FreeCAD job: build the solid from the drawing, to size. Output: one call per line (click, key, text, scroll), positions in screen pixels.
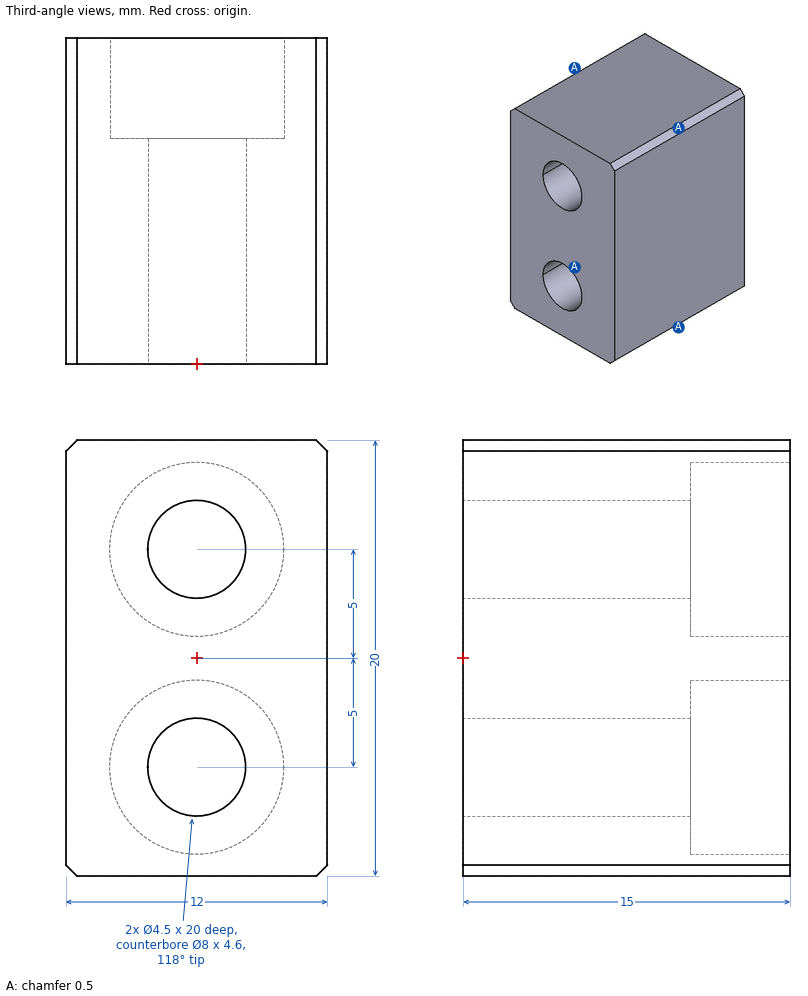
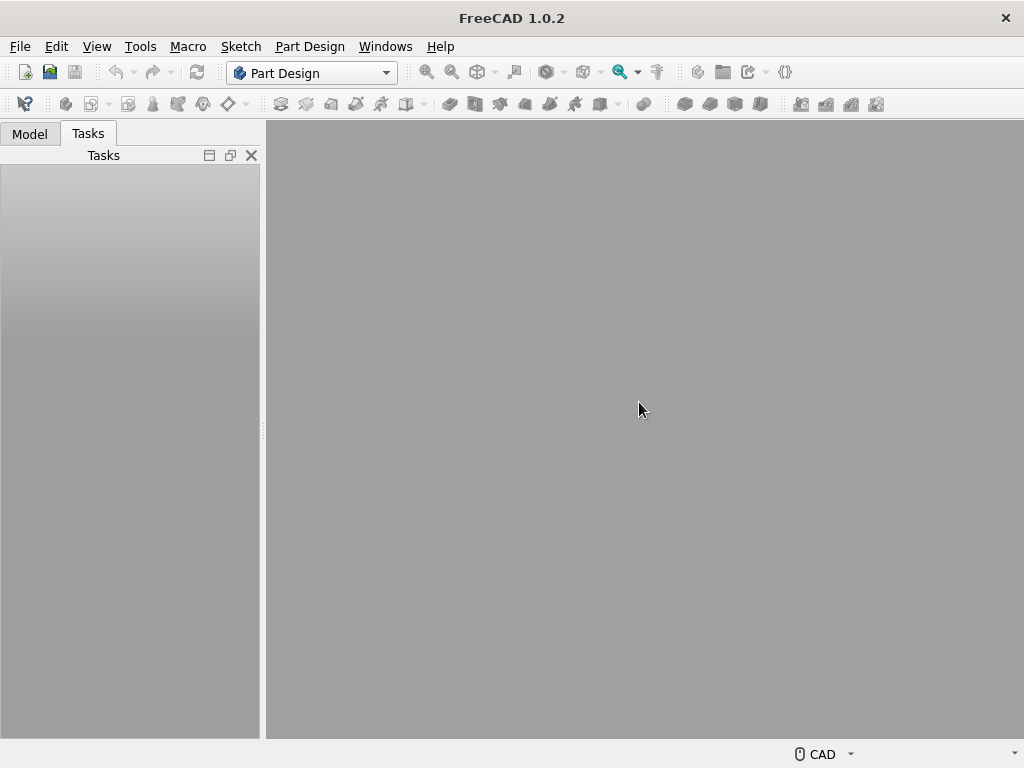
click(25, 72)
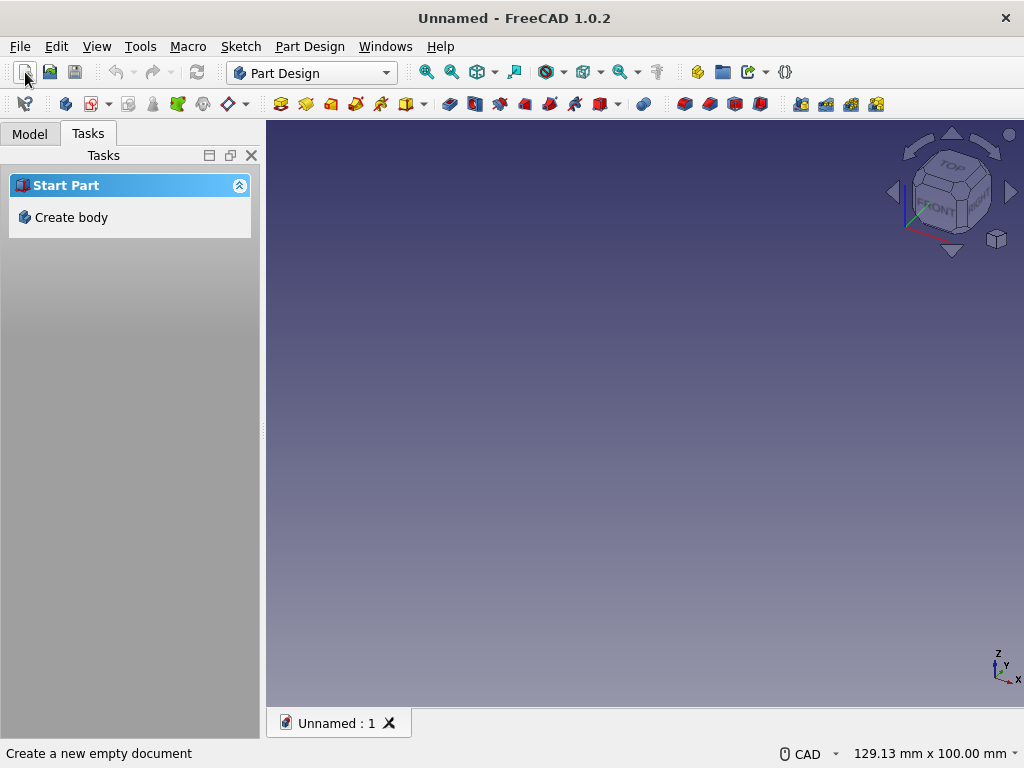
click(90, 104)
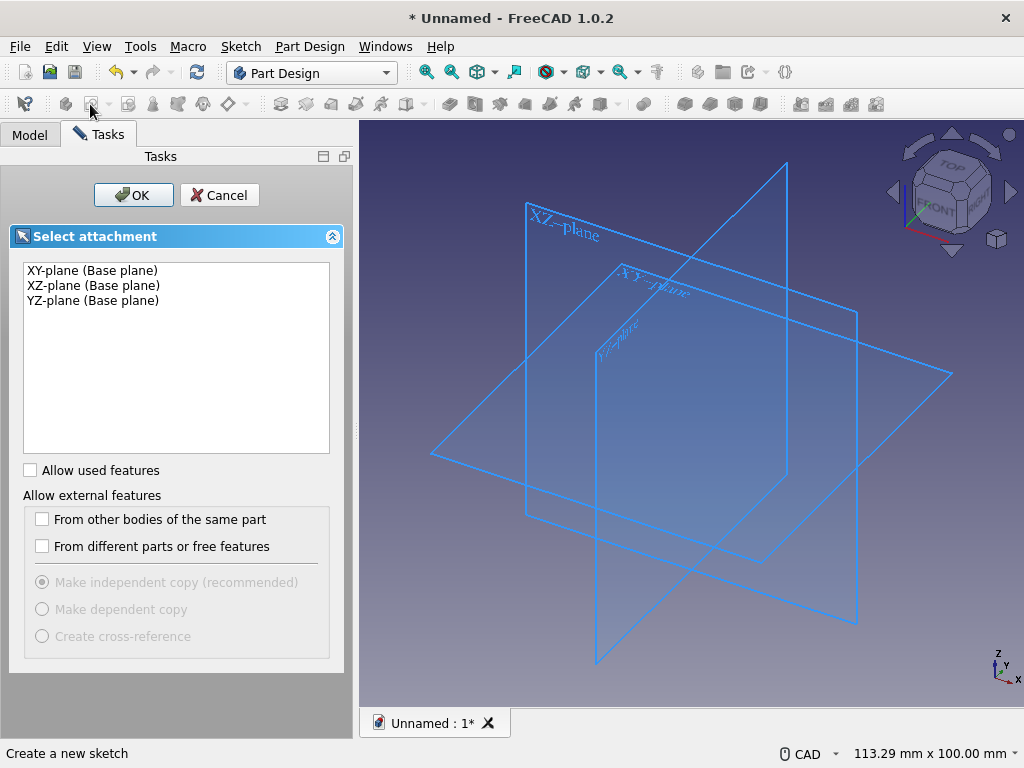
click(84, 286)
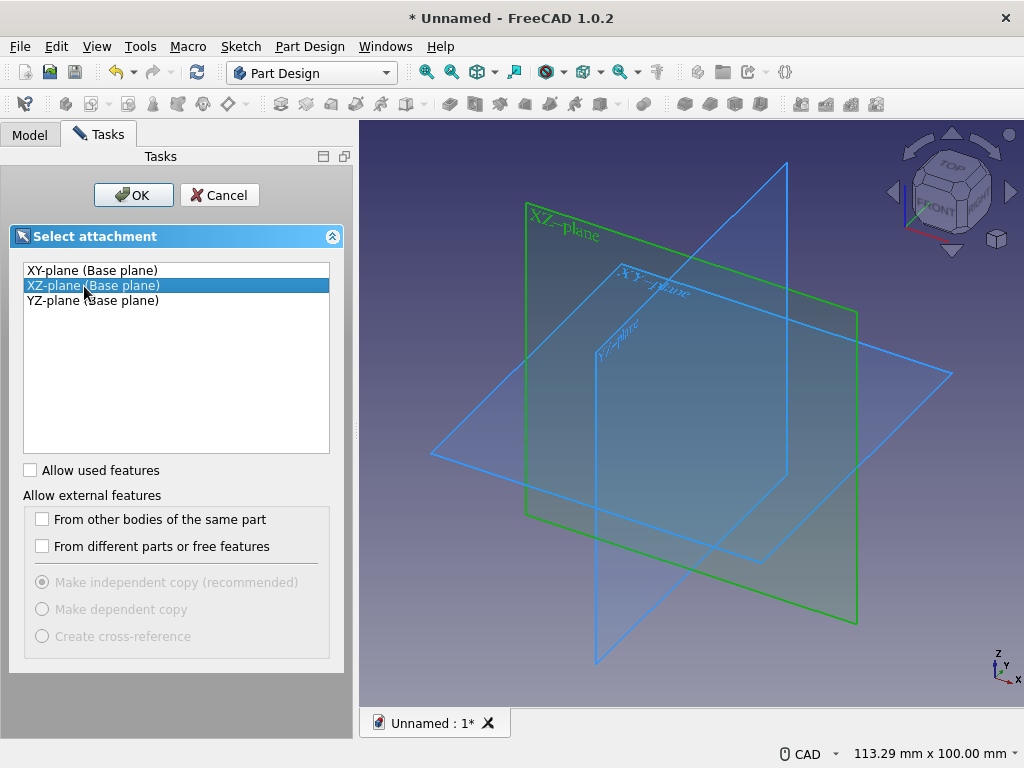
click(134, 195)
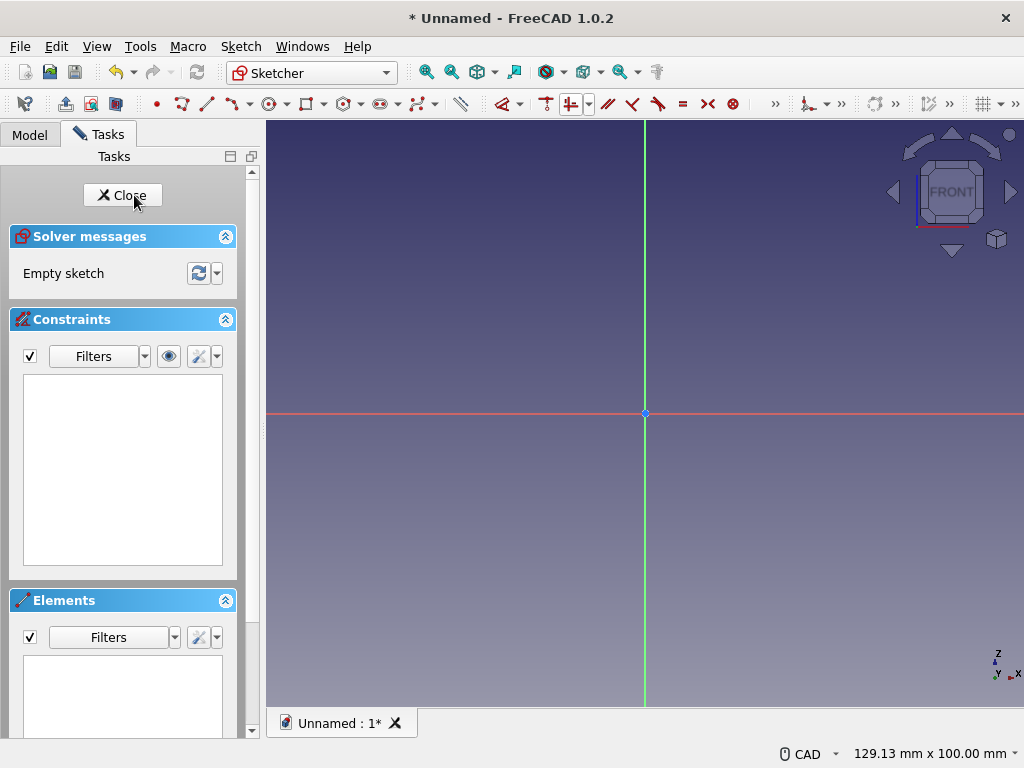
scroll(675, 414, up, 6)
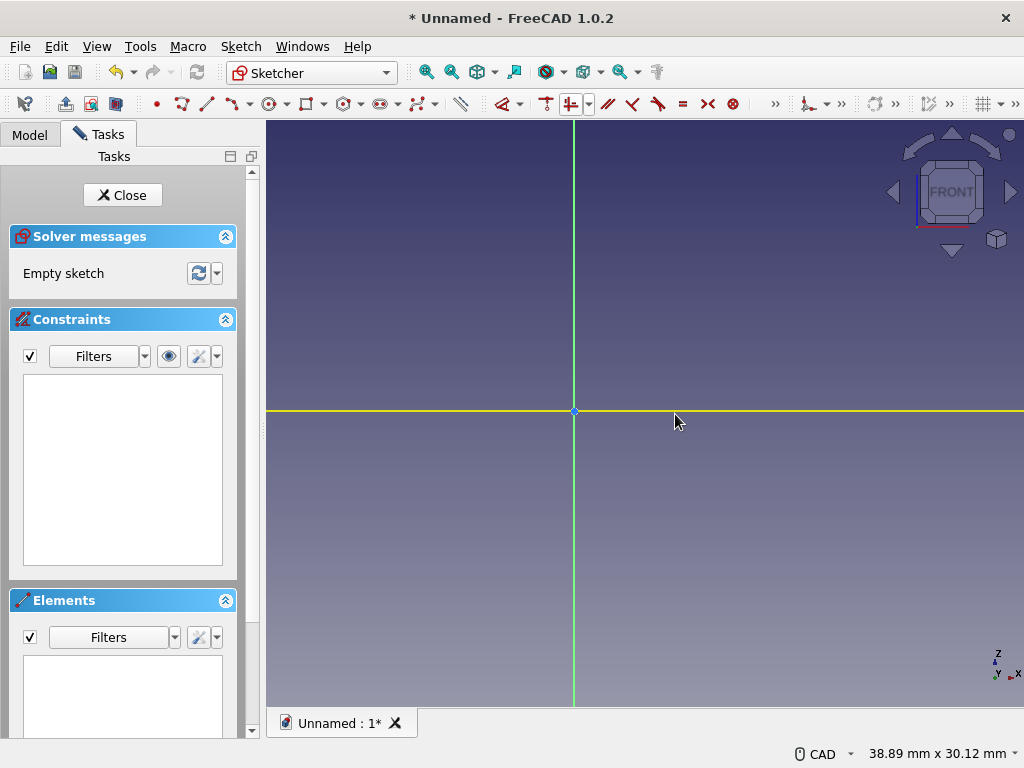
click(324, 104)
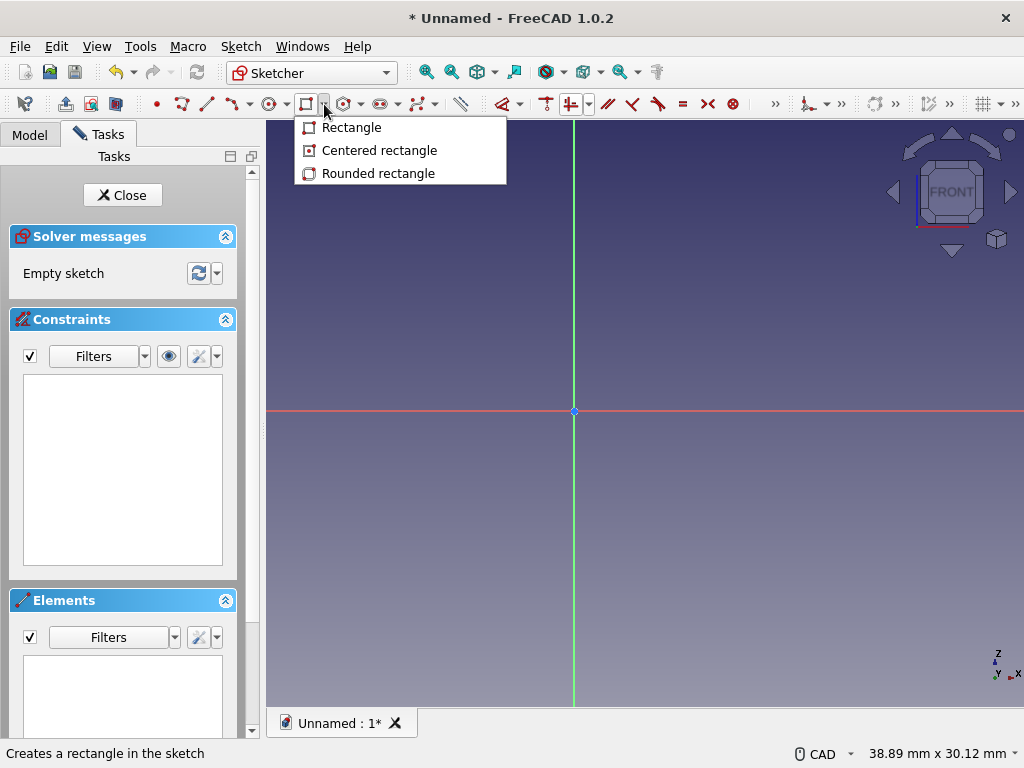
click(400, 150)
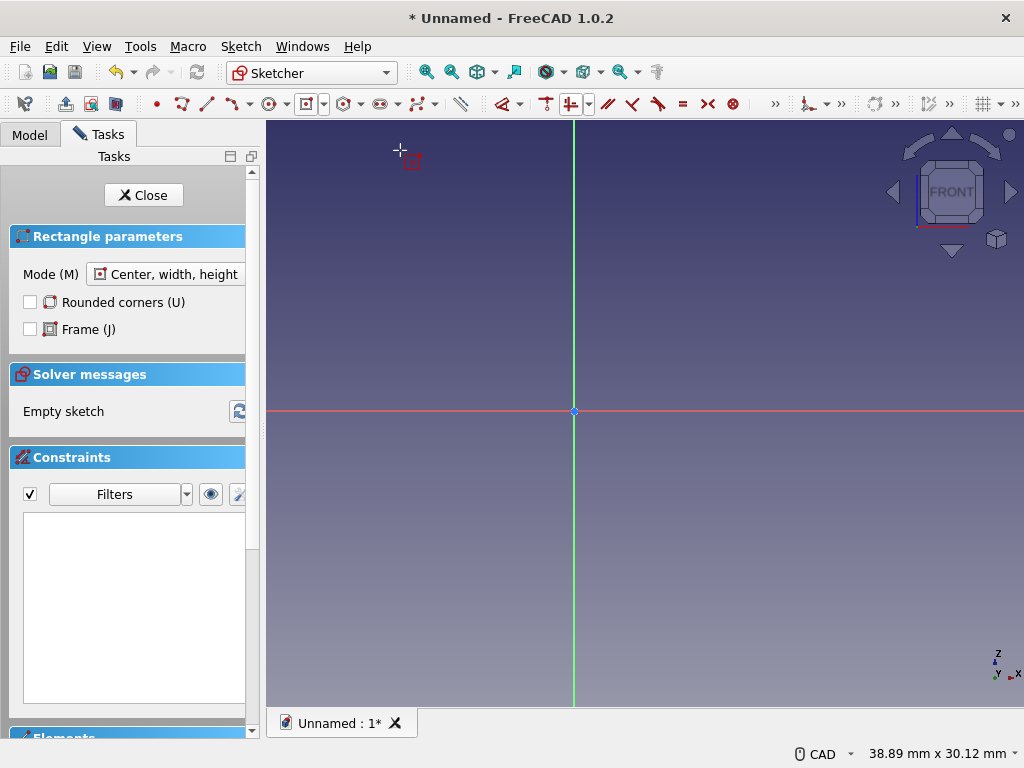
click(574, 411)
click(691, 216)
key(Escape)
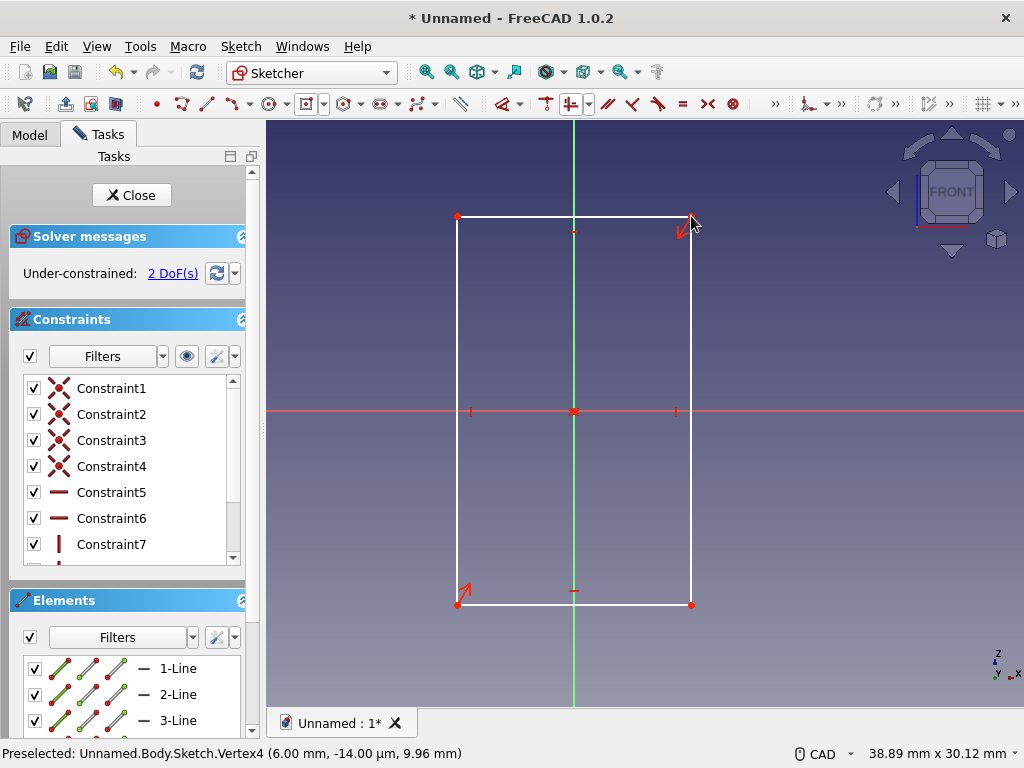
click(527, 605)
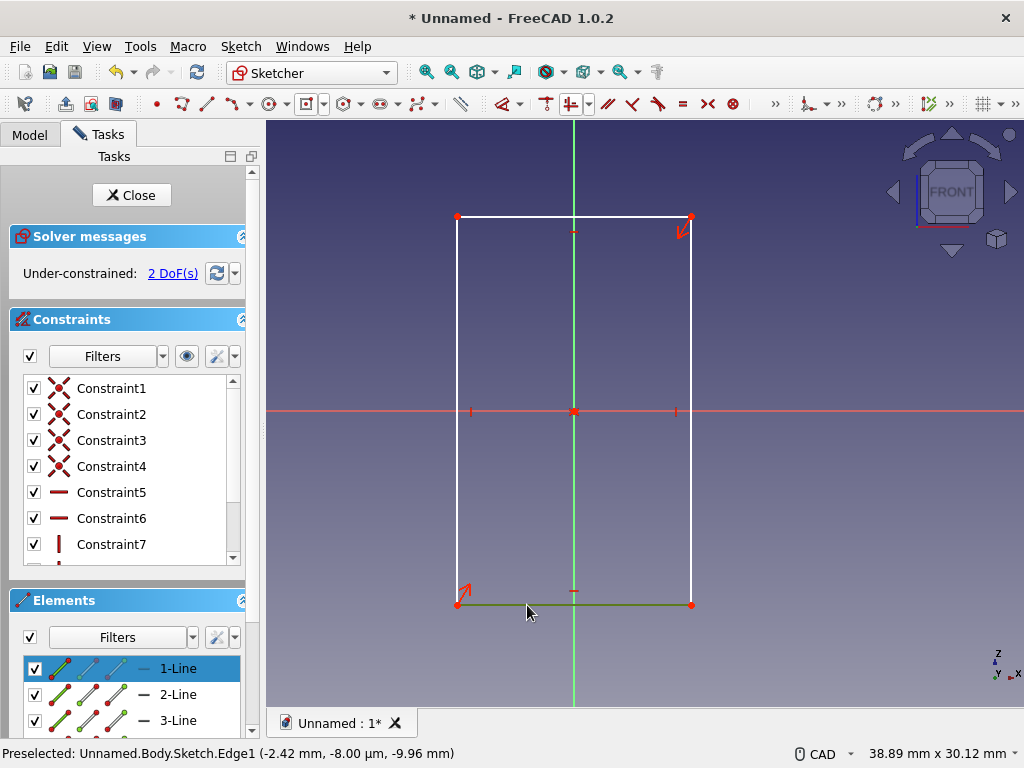
key(l)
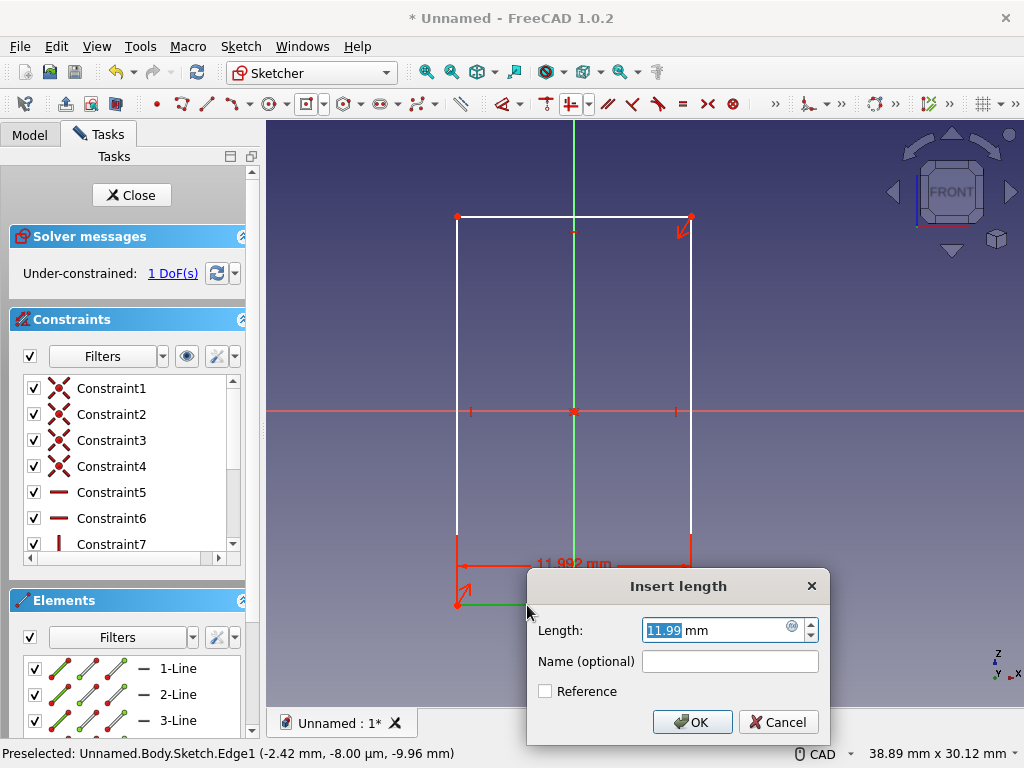
text(12)
key(Return)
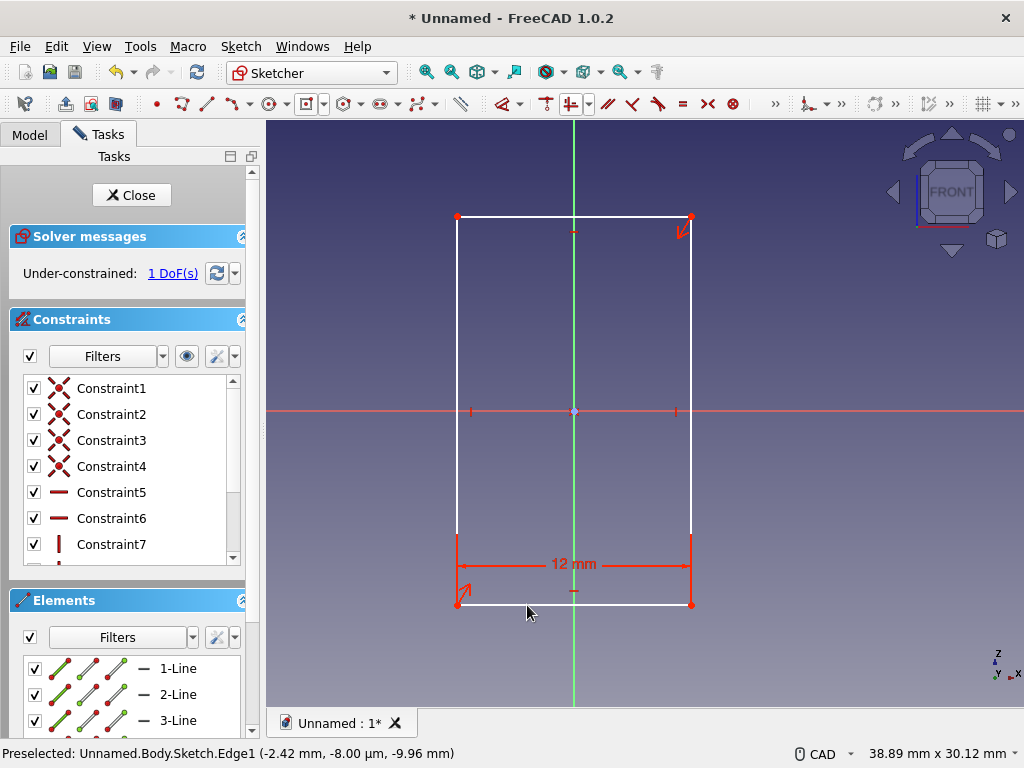
click(691, 489)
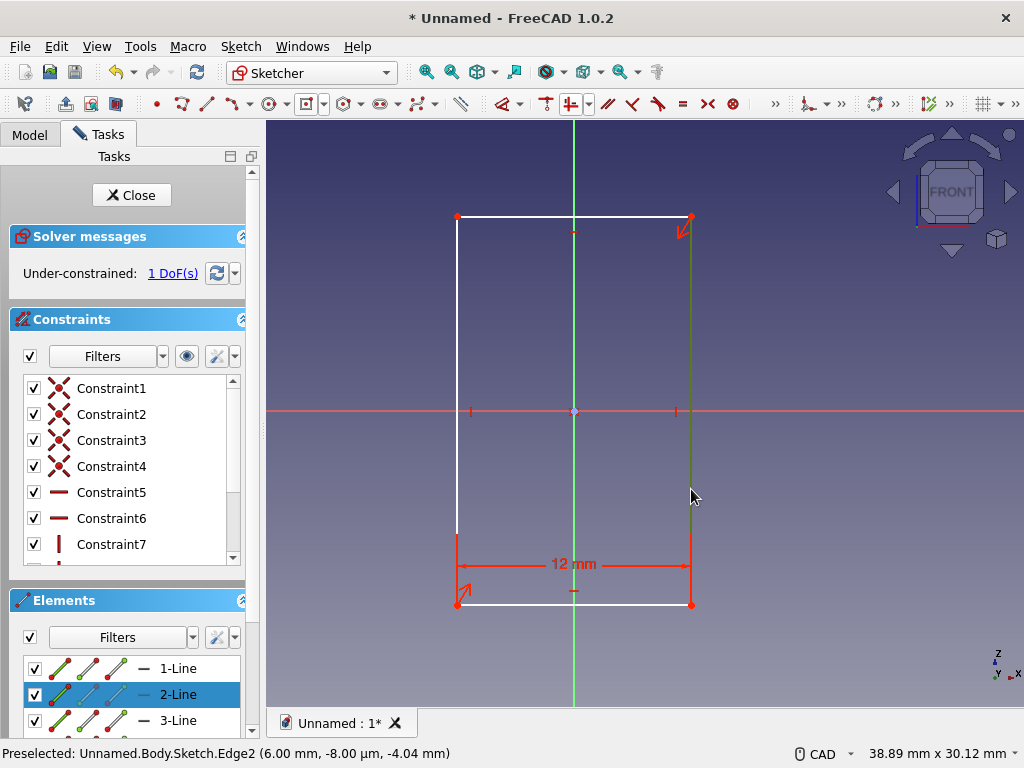
key(i)